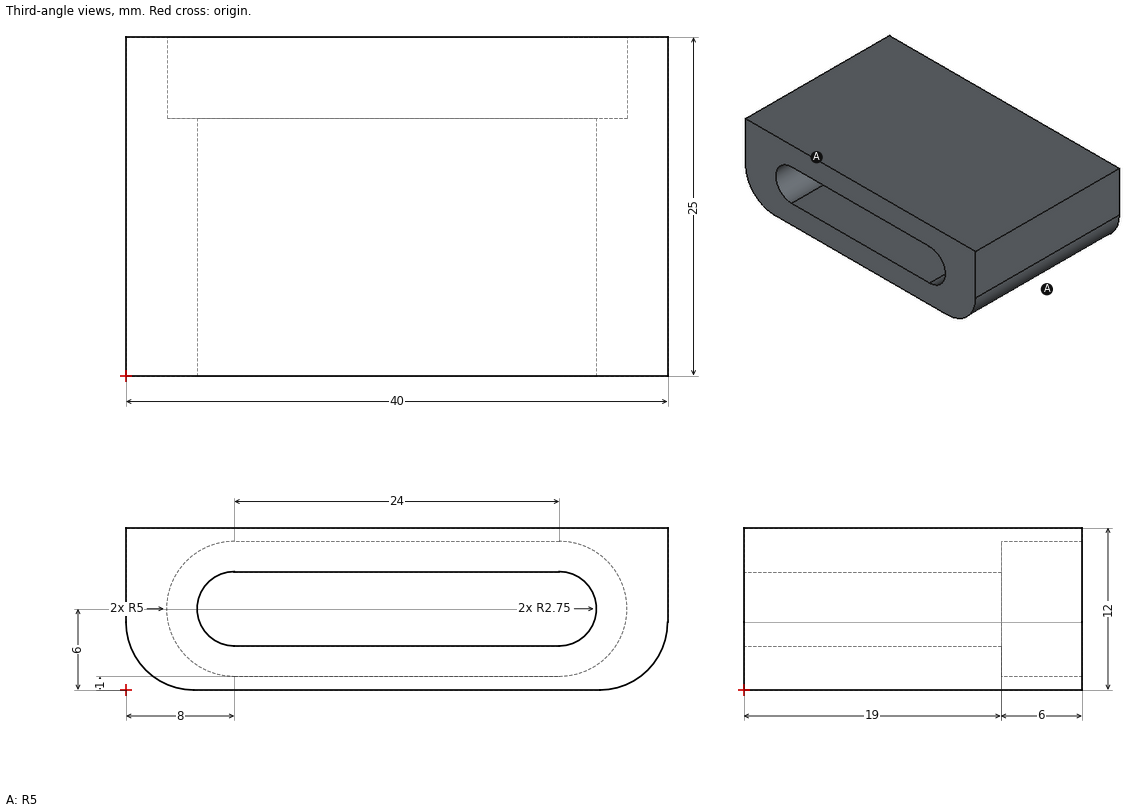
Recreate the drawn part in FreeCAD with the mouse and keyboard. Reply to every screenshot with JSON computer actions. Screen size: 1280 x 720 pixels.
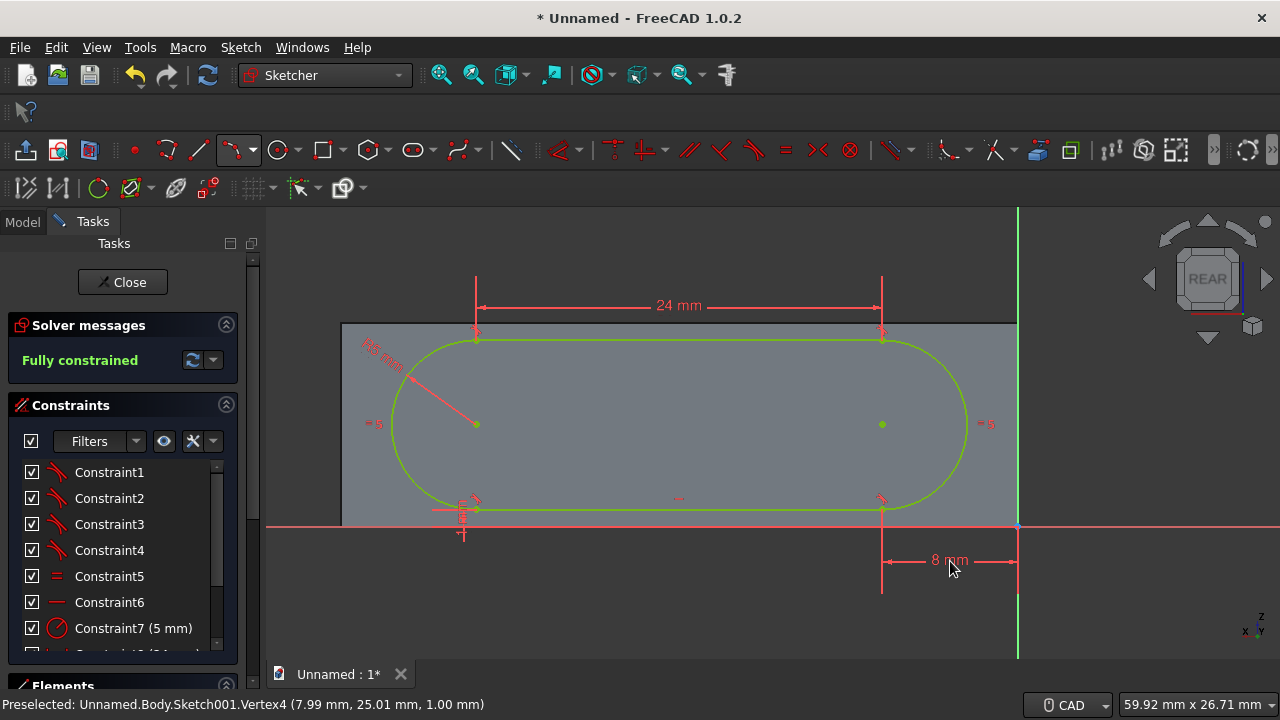
{"action": "left_click", "coordinate": [123, 282]}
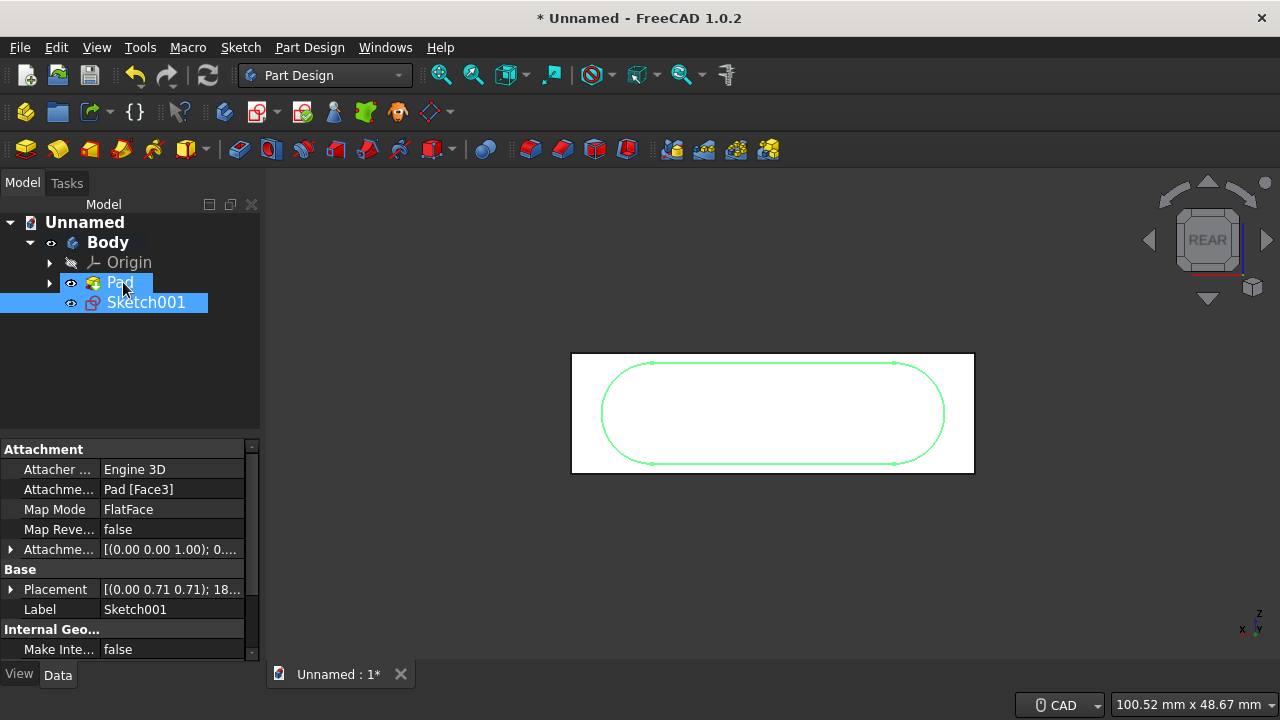
{"action": "left_click", "coordinate": [240, 150]}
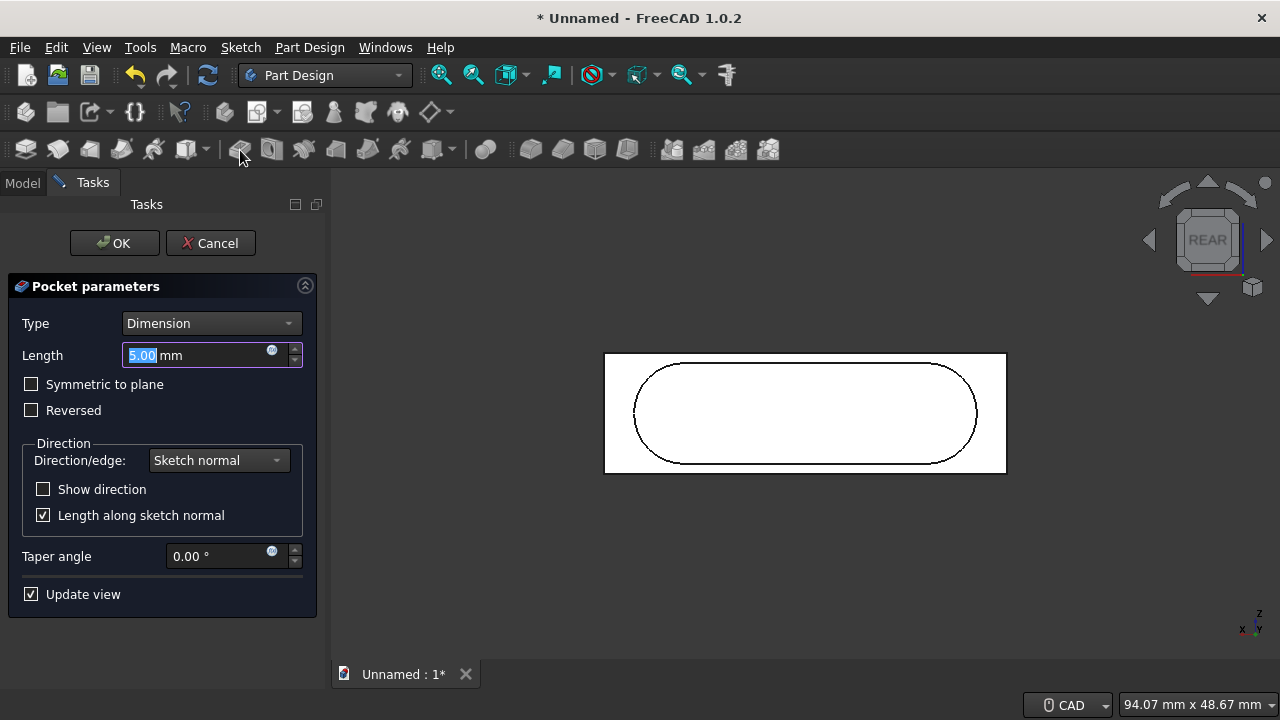
{"action": "type", "text": "6"}
{"action": "key", "text": "Tab"}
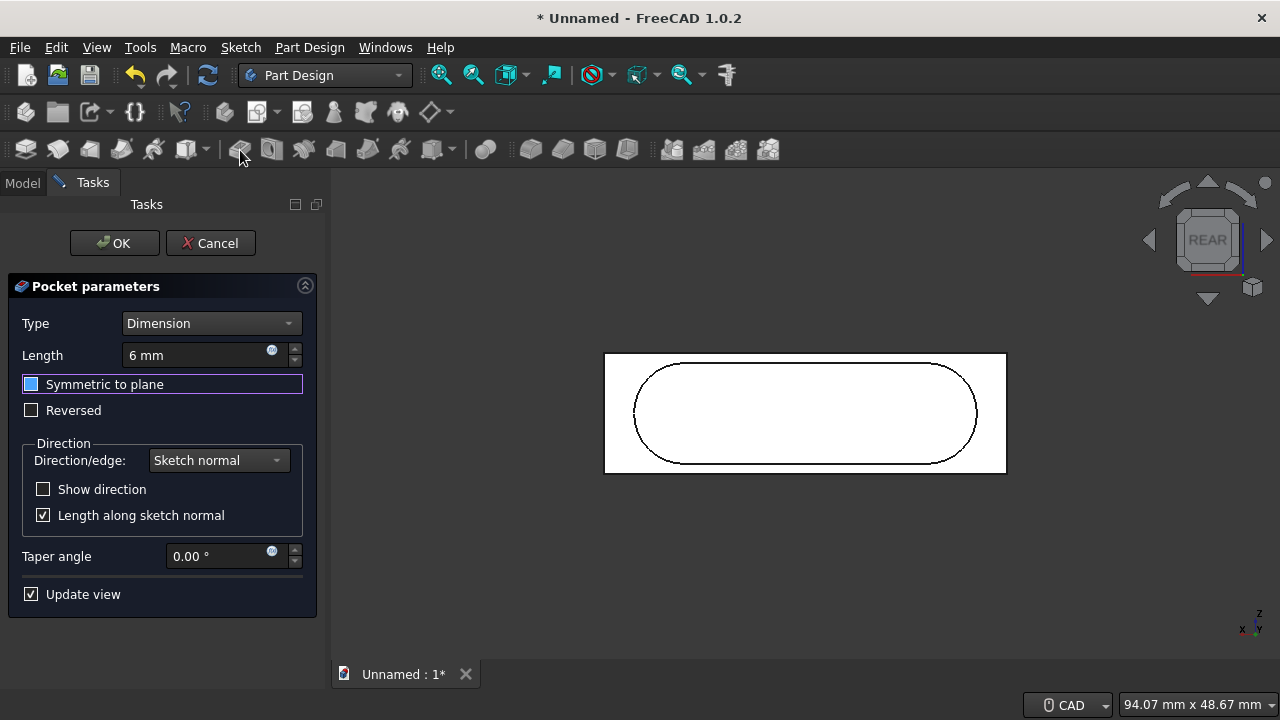
{"action": "left_click", "coordinate": [115, 243]}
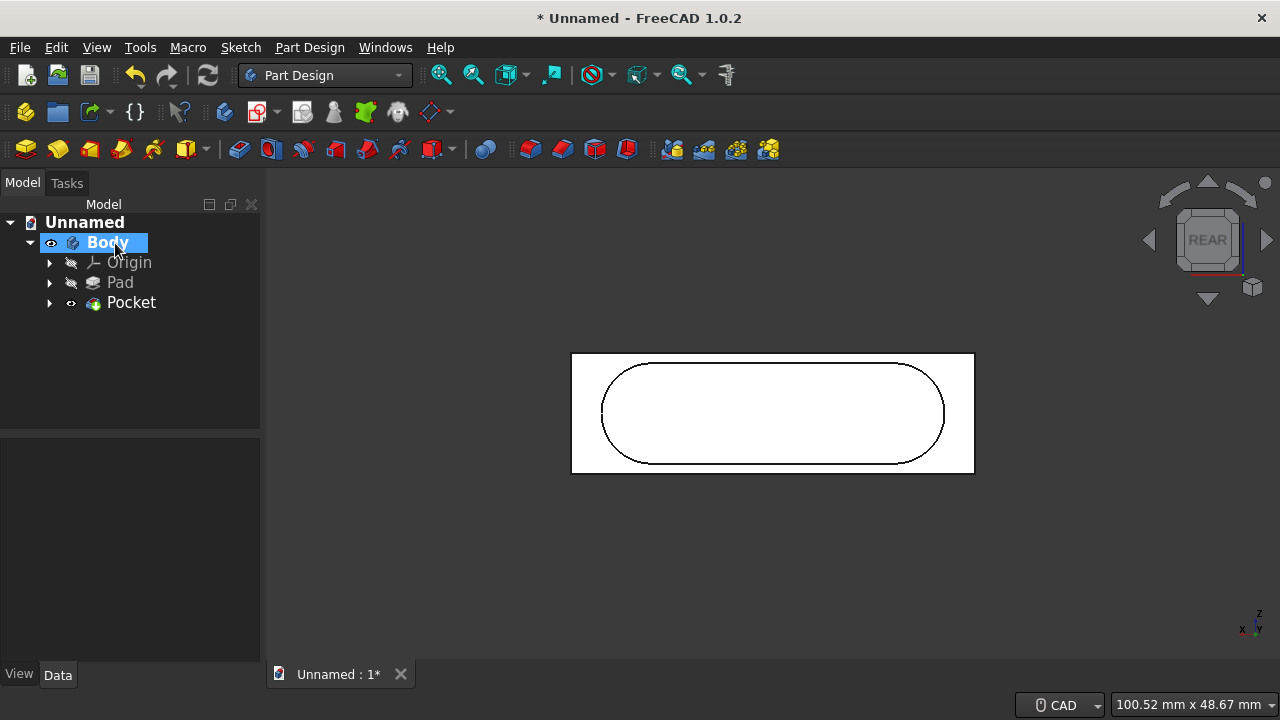
{"action": "key", "text": "v f"}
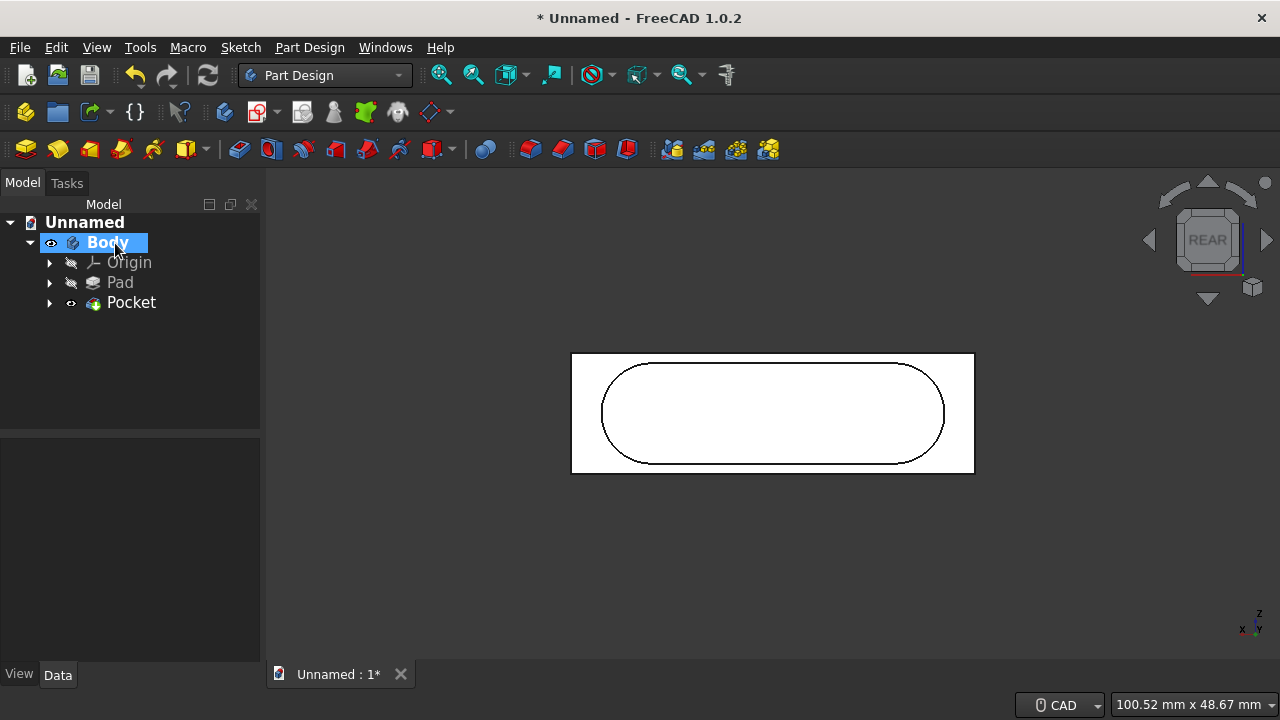
{"action": "left_click", "coordinate": [675, 412]}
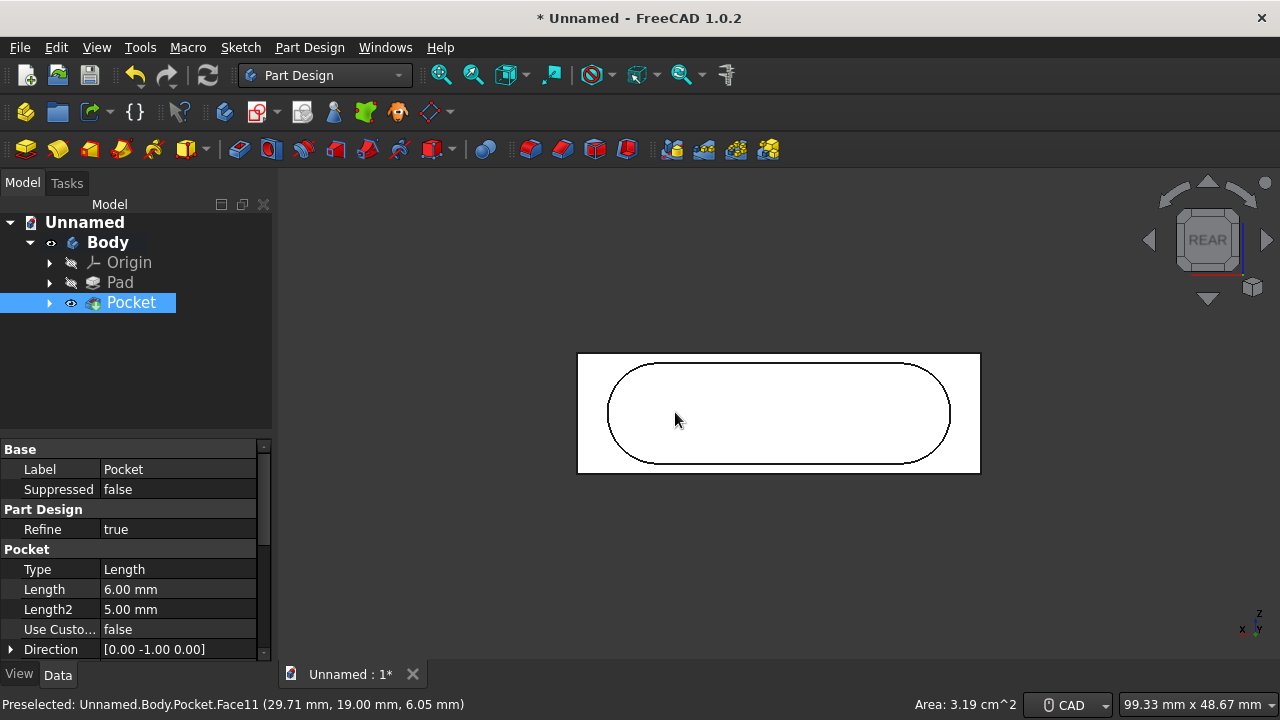
{"action": "left_click", "coordinate": [258, 112]}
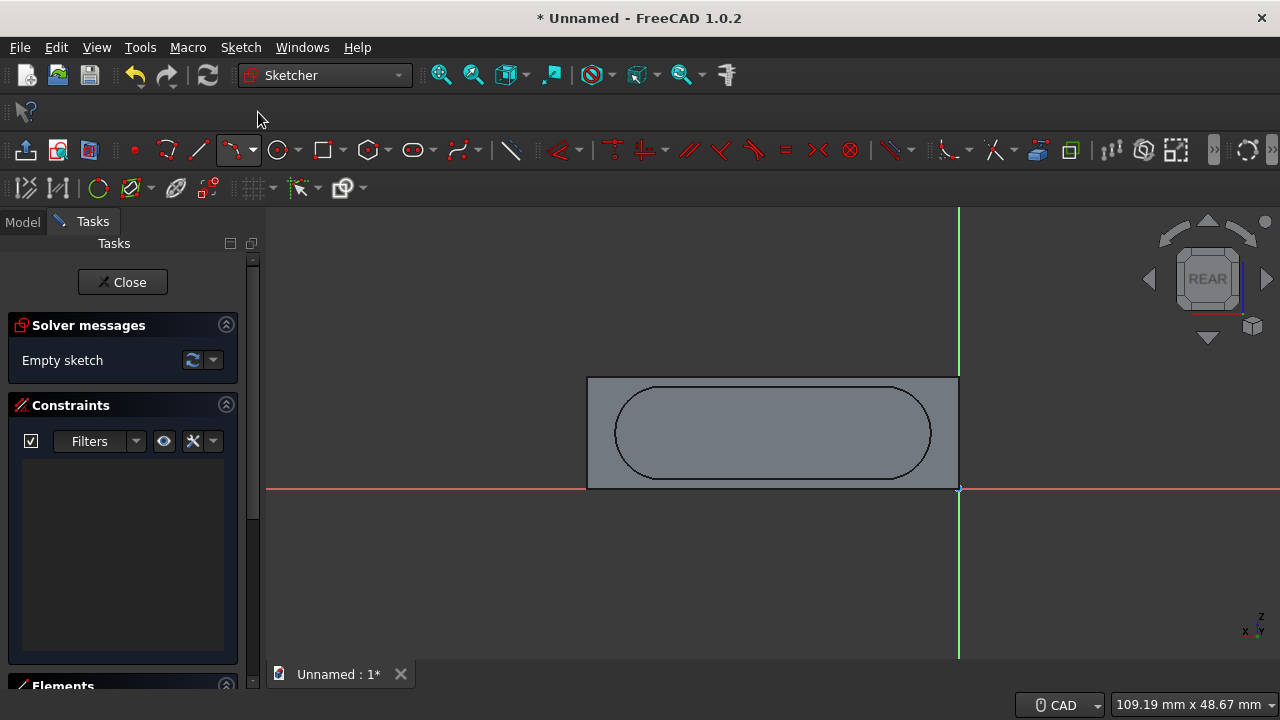
{"action": "key", "text": "q s"}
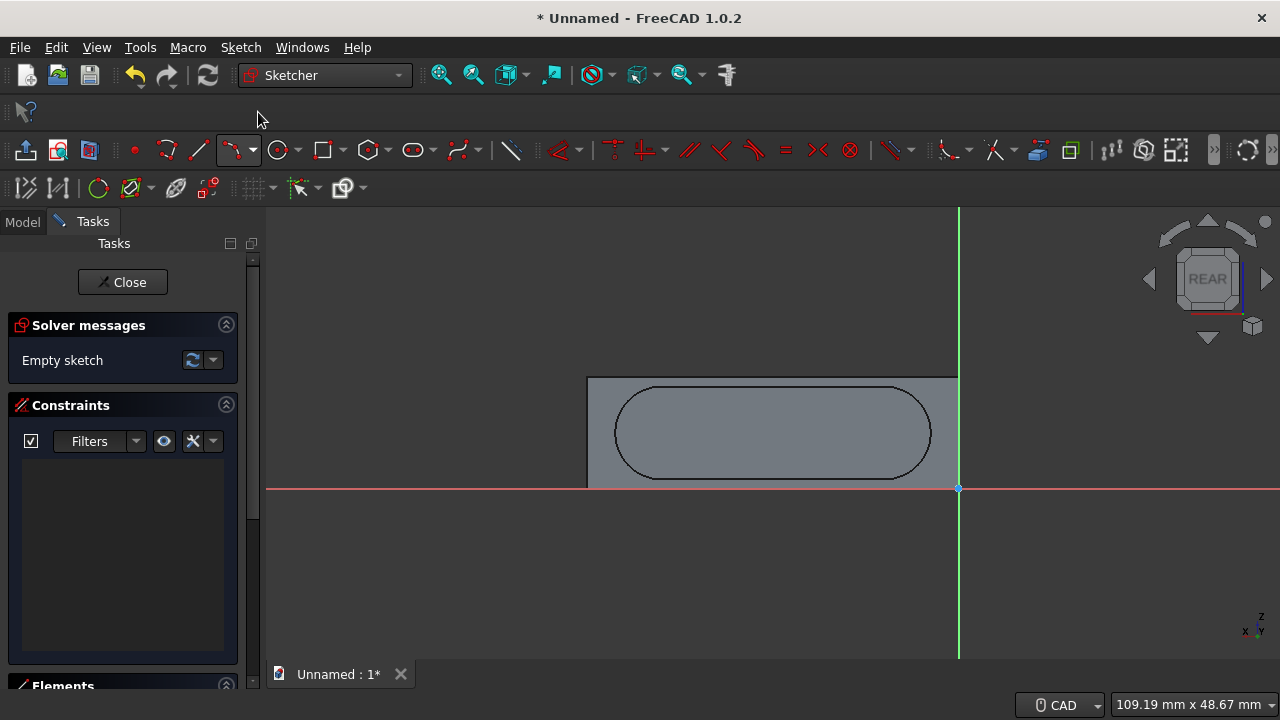
{"action": "scroll", "coordinate": [910, 466], "scroll_direction": "up", "scroll_amount": 3}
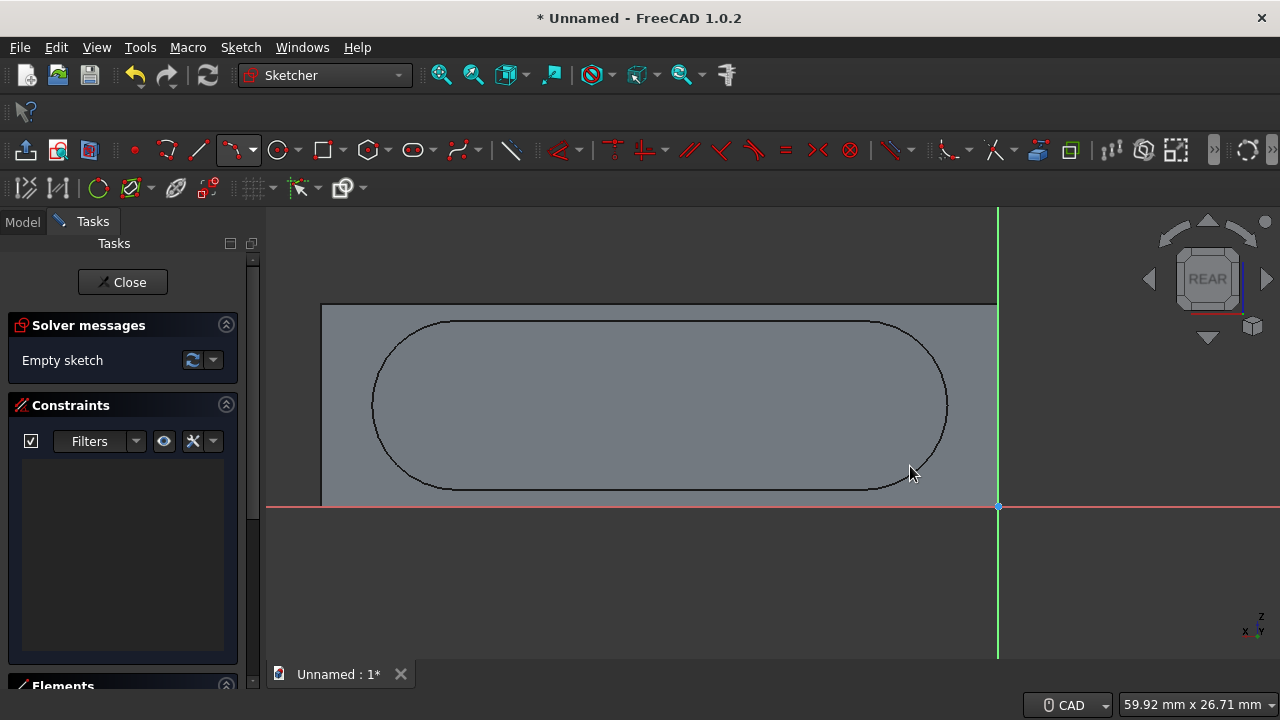
{"action": "key", "text": "g s"}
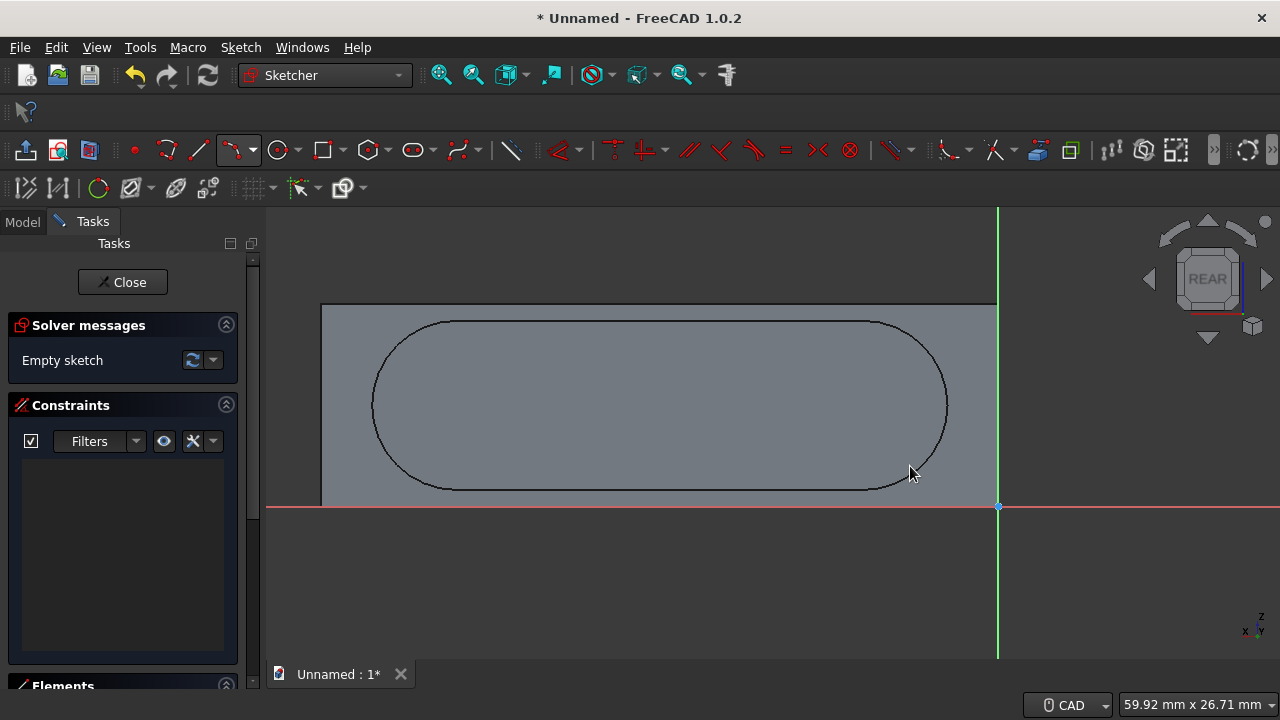
{"action": "left_click", "coordinate": [457, 405]}